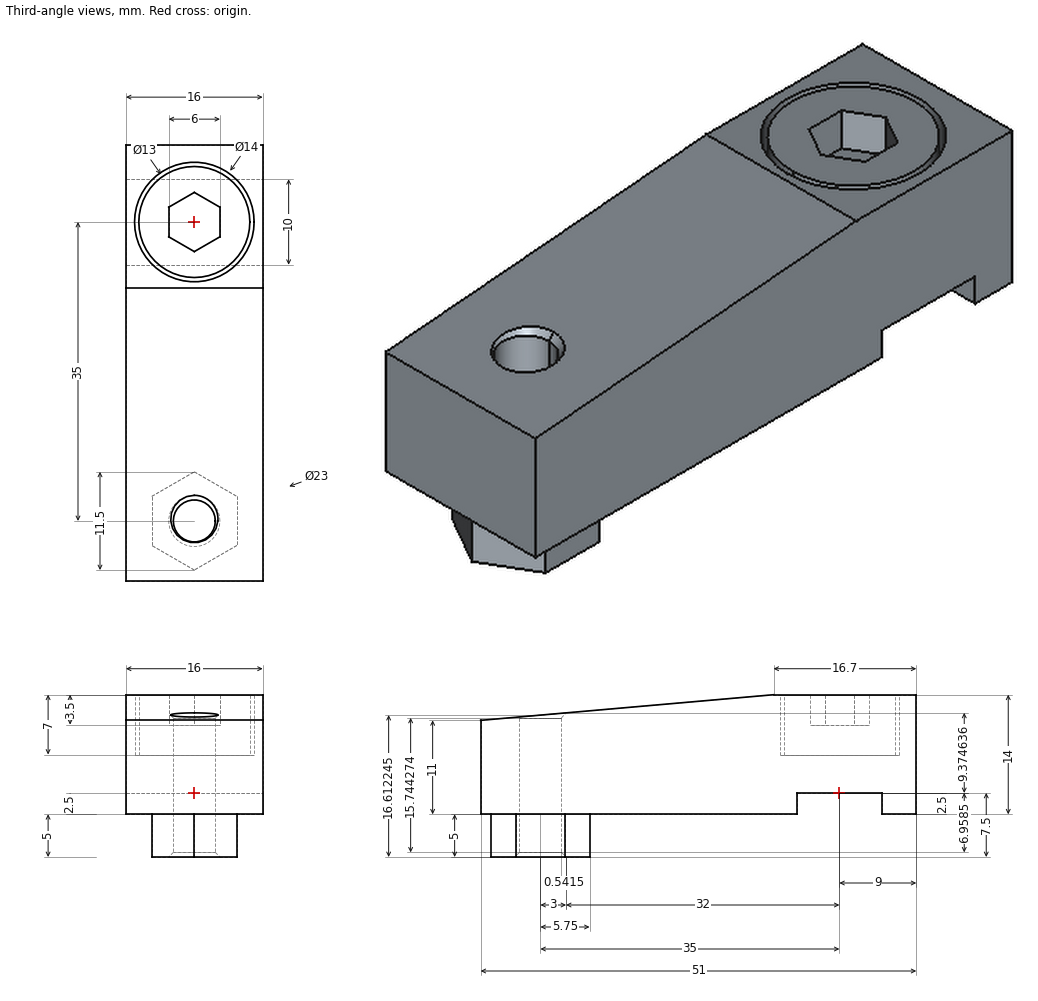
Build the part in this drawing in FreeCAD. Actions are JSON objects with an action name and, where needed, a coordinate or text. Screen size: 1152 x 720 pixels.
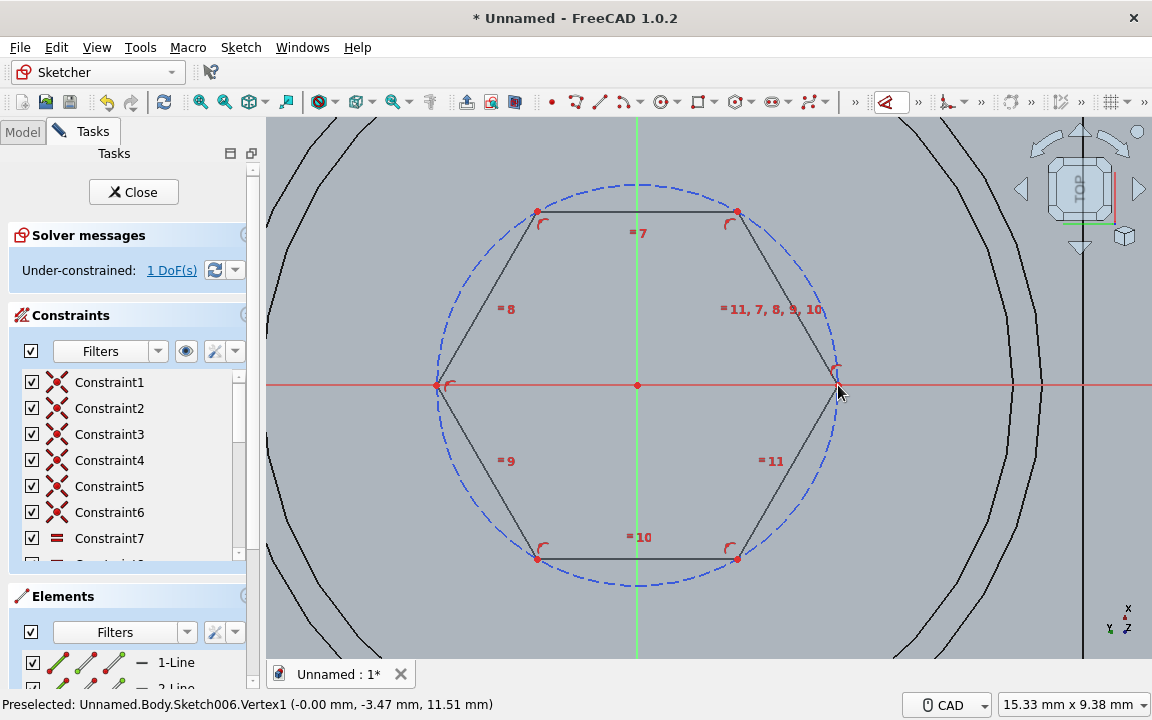
{"action": "left_click", "coordinate": [537, 559]}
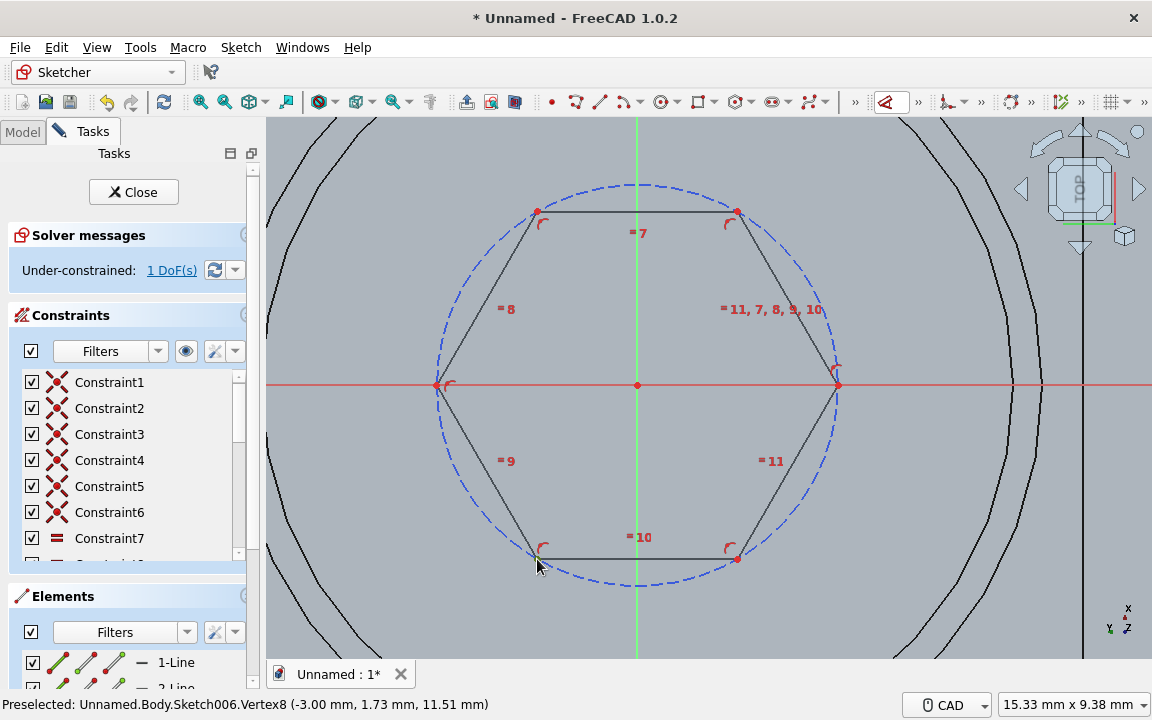
{"action": "left_click", "coordinate": [738, 212]}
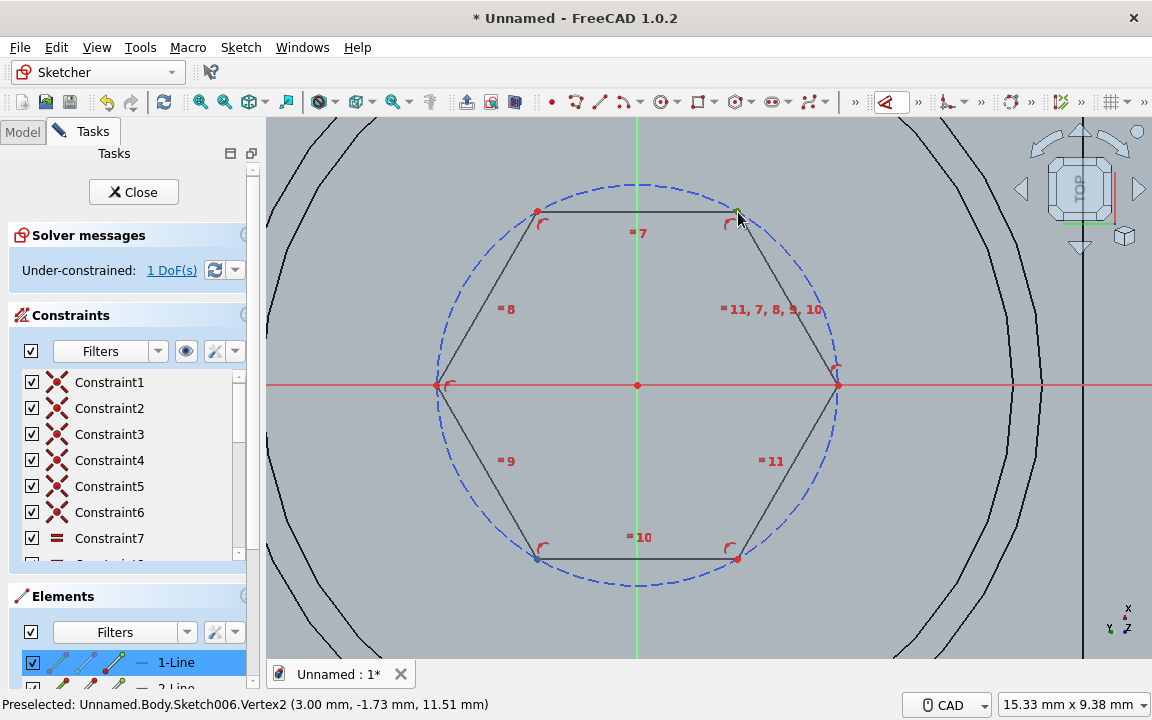
{"action": "left_click", "coordinate": [904, 102]}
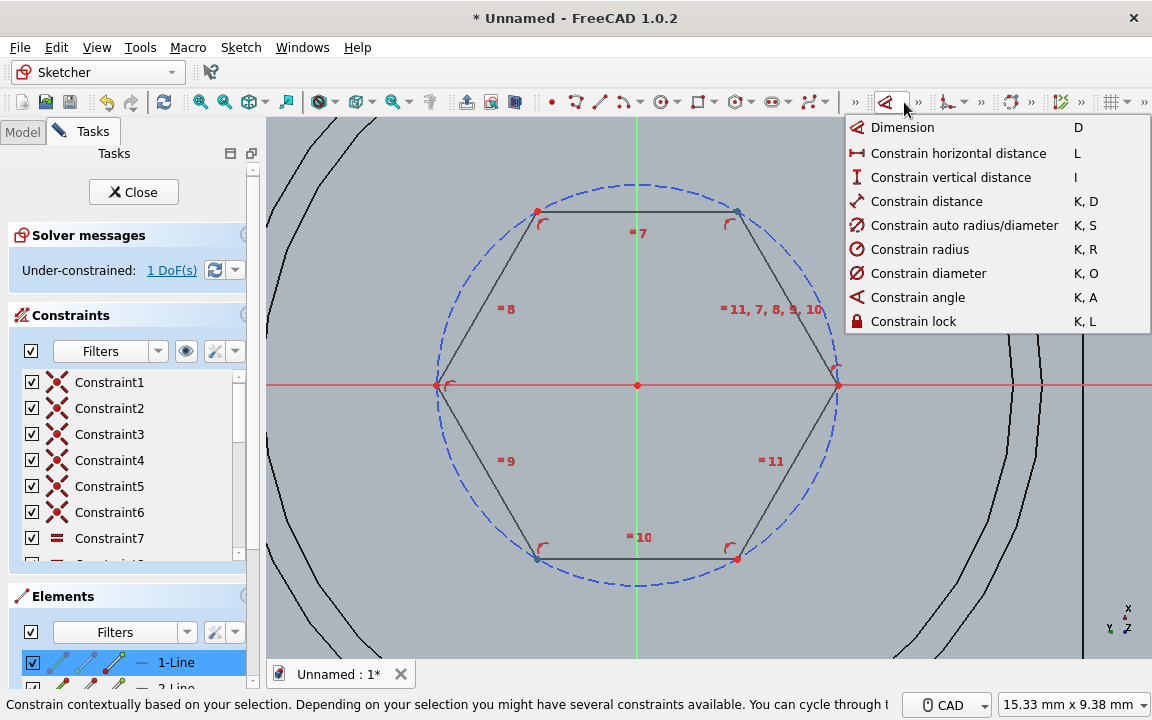
{"action": "left_click", "coordinate": [998, 177]}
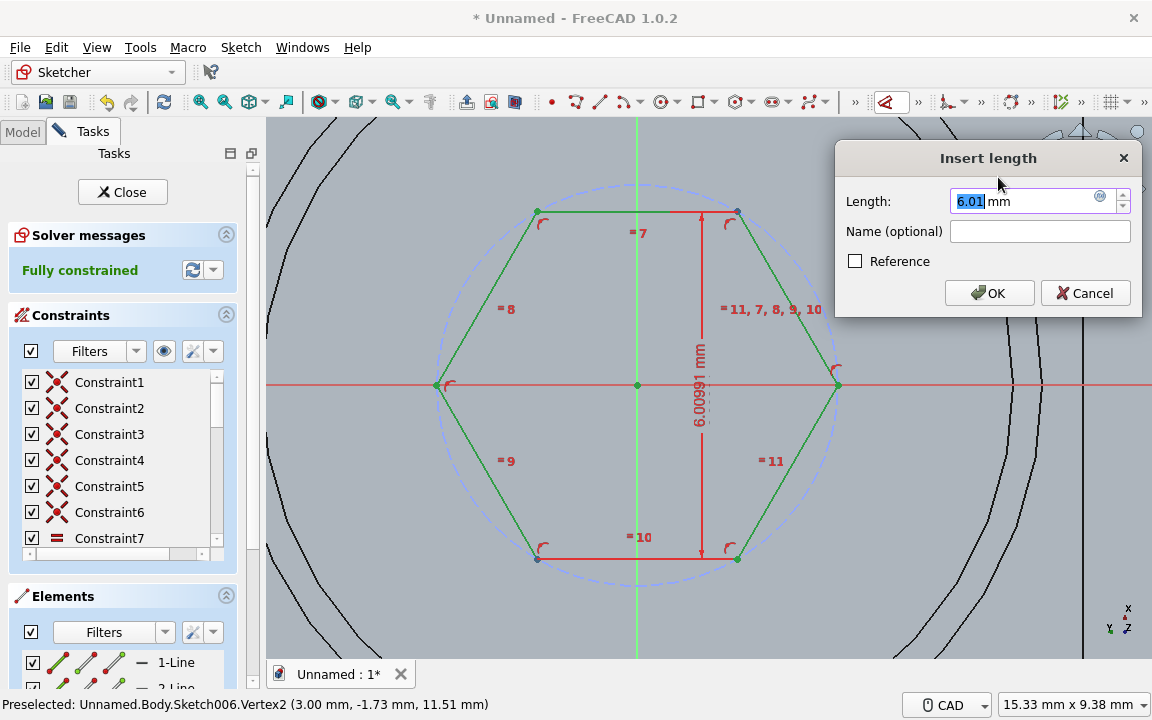
{"action": "type", "text": "6"}
{"action": "key", "text": "Return"}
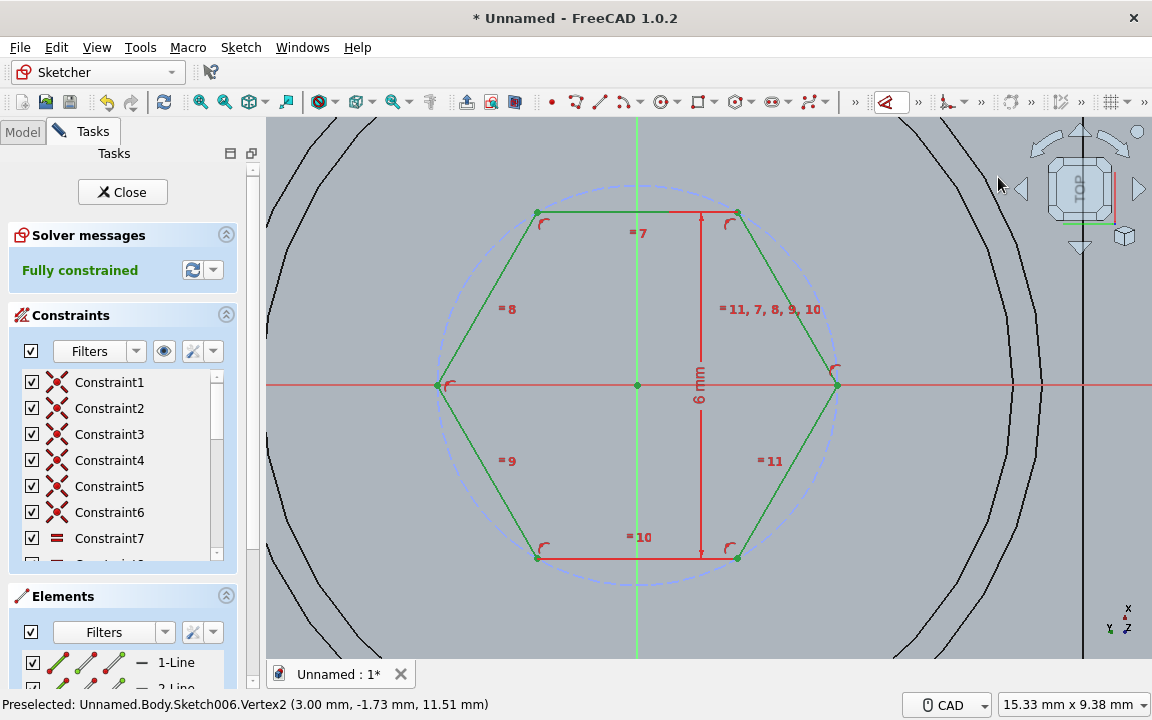
{"action": "left_click", "coordinate": [123, 192]}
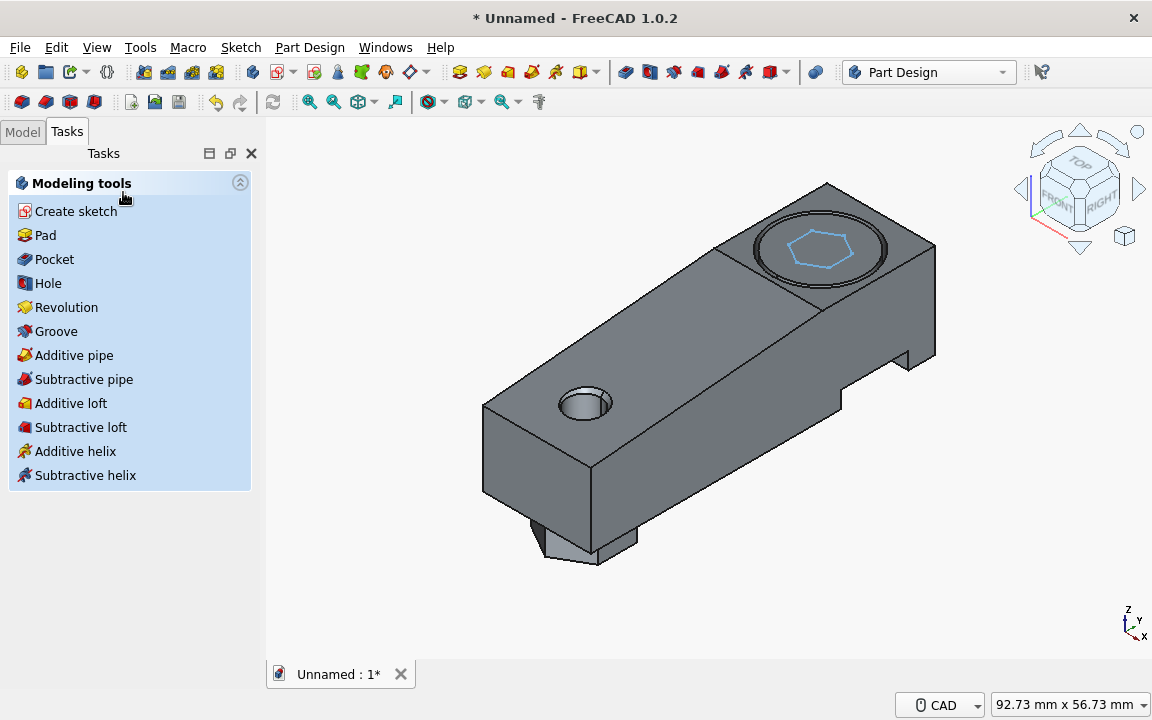
{"action": "left_click", "coordinate": [626, 72]}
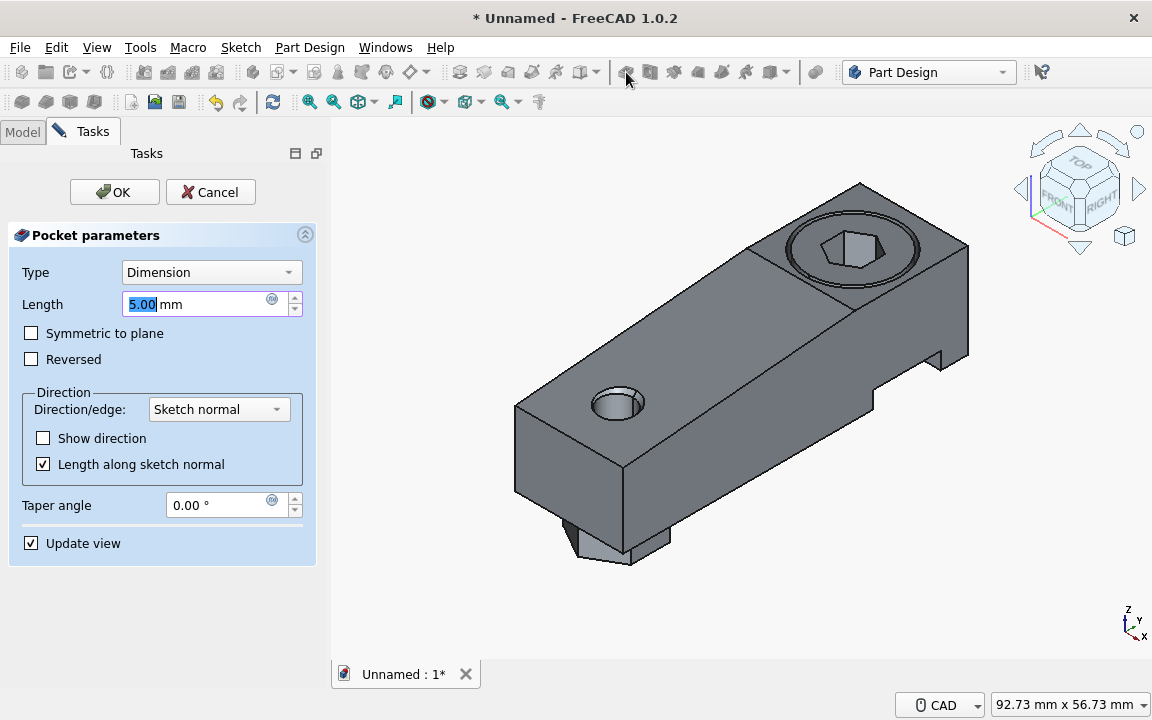
{"action": "type", "text": "3.5"}
{"action": "key", "text": "Tab"}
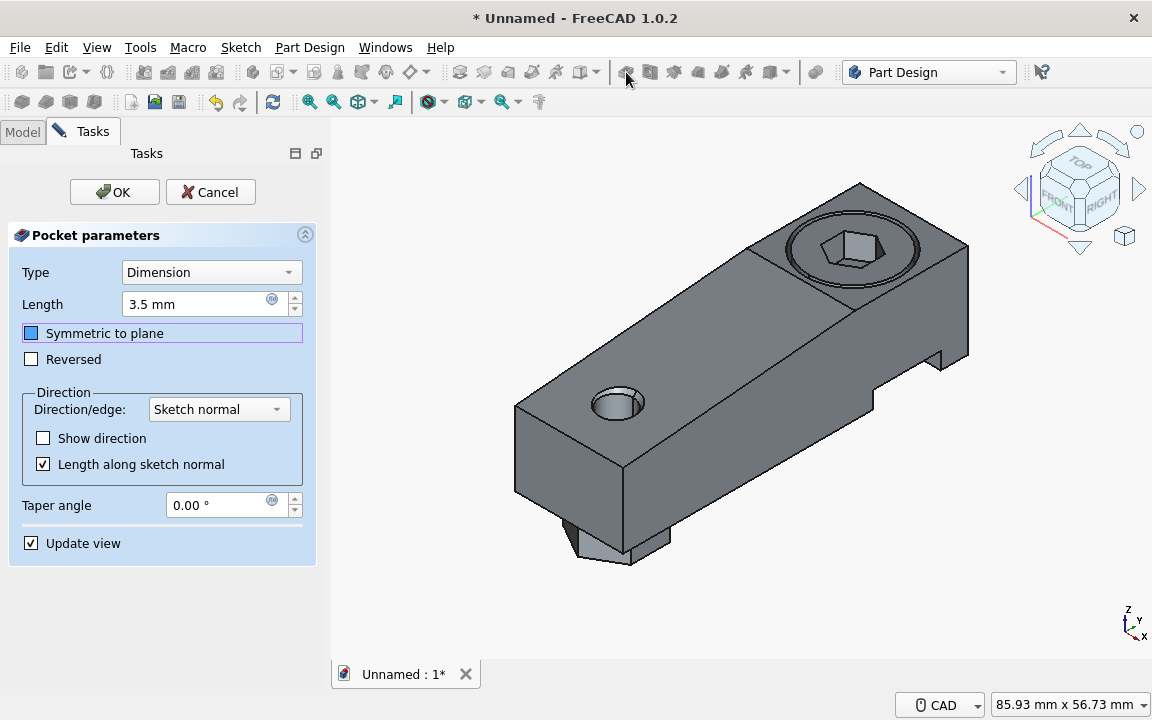
{"action": "left_click", "coordinate": [115, 192]}